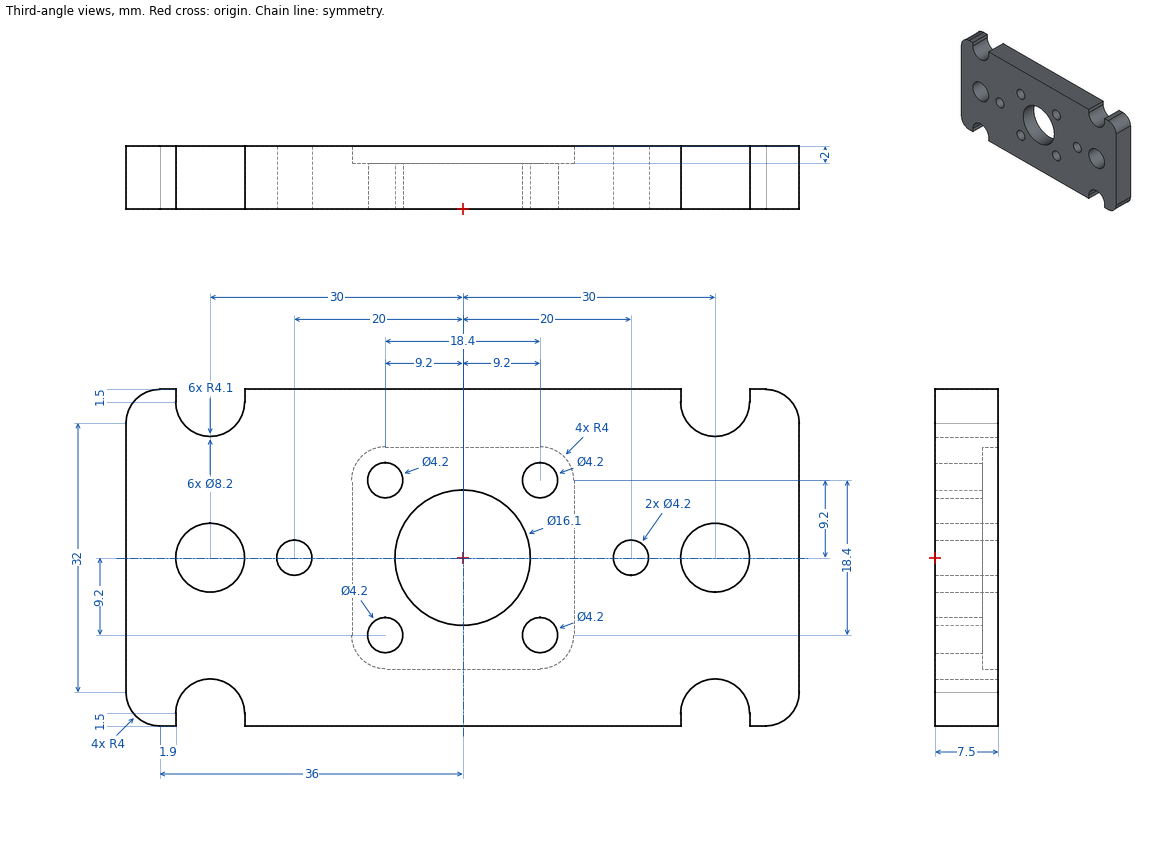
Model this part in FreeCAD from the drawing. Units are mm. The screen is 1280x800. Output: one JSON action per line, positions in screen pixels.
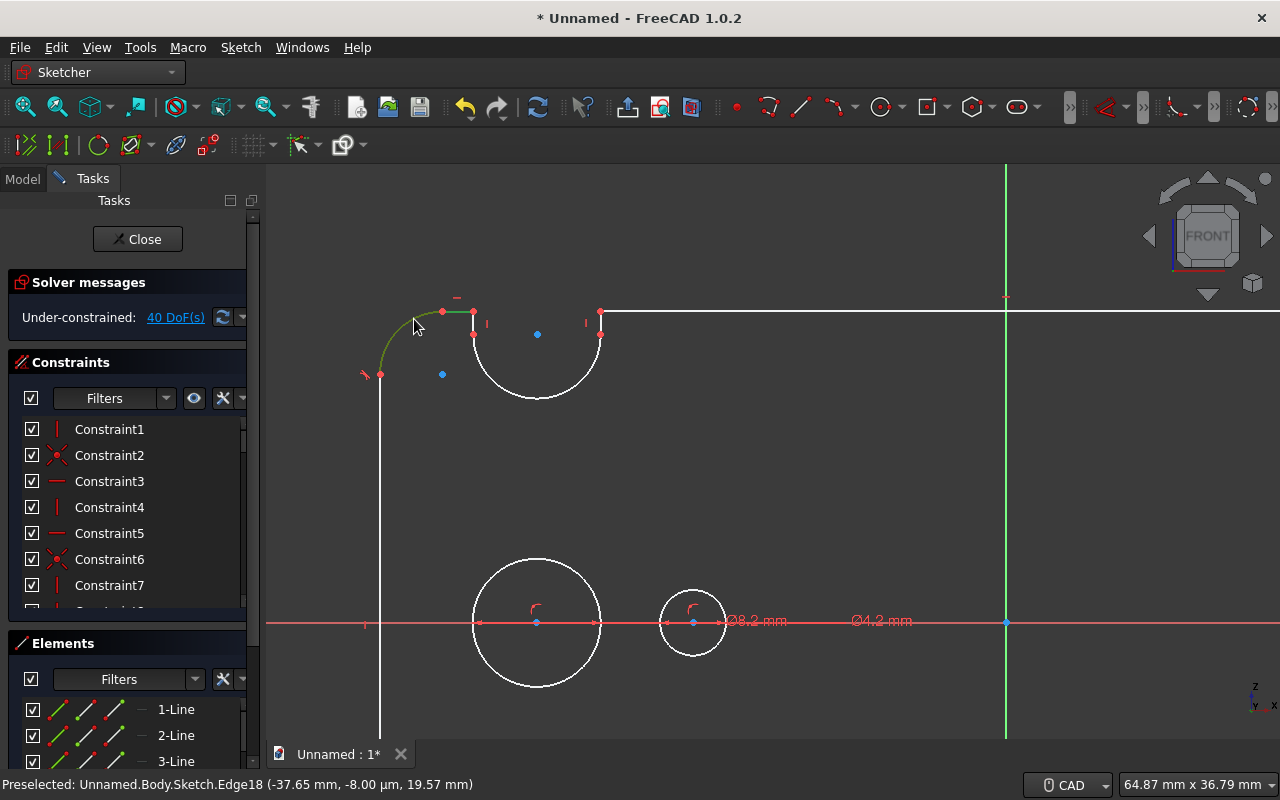
{"action": "key", "text": "t"}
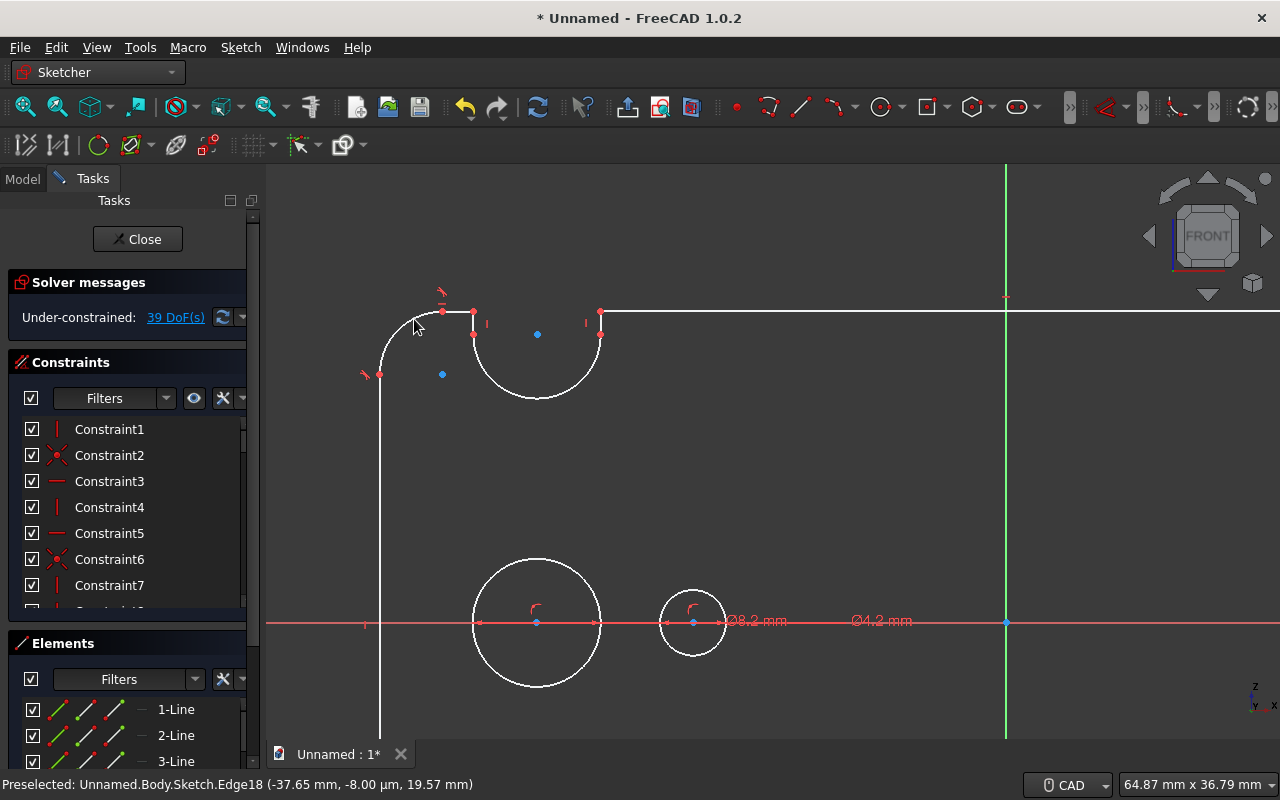
{"action": "scroll", "coordinate": [473, 321], "scroll_direction": "up", "scroll_amount": 3}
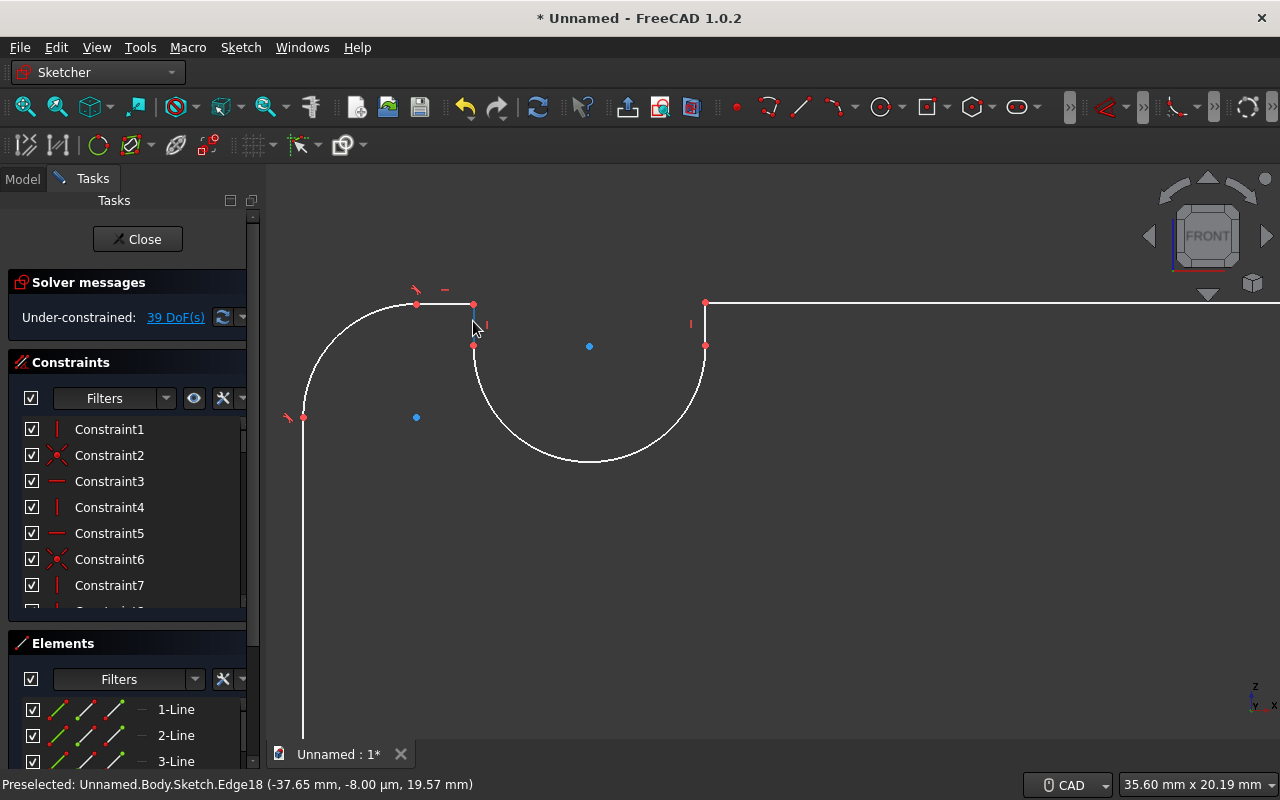
{"action": "left_click", "coordinate": [474, 320]}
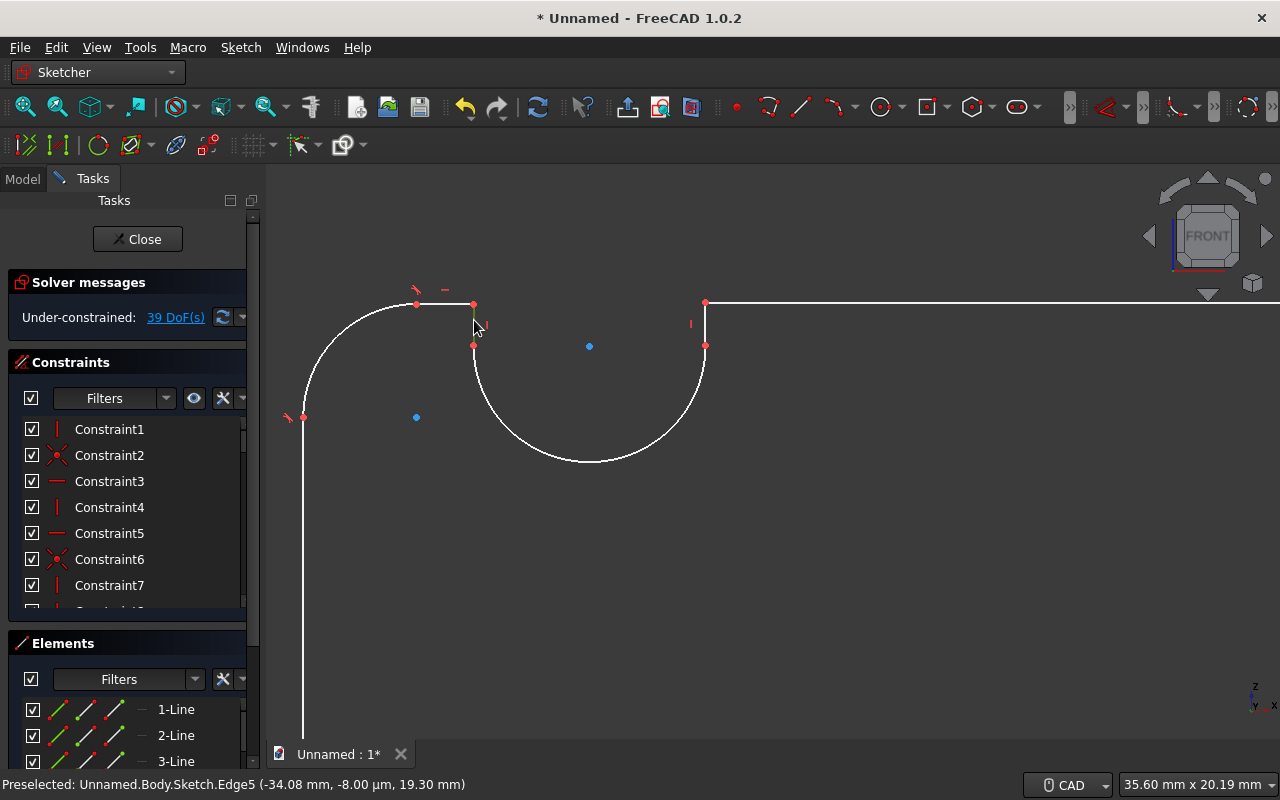
{"action": "scroll", "coordinate": [462, 314], "scroll_direction": "down", "scroll_amount": 7}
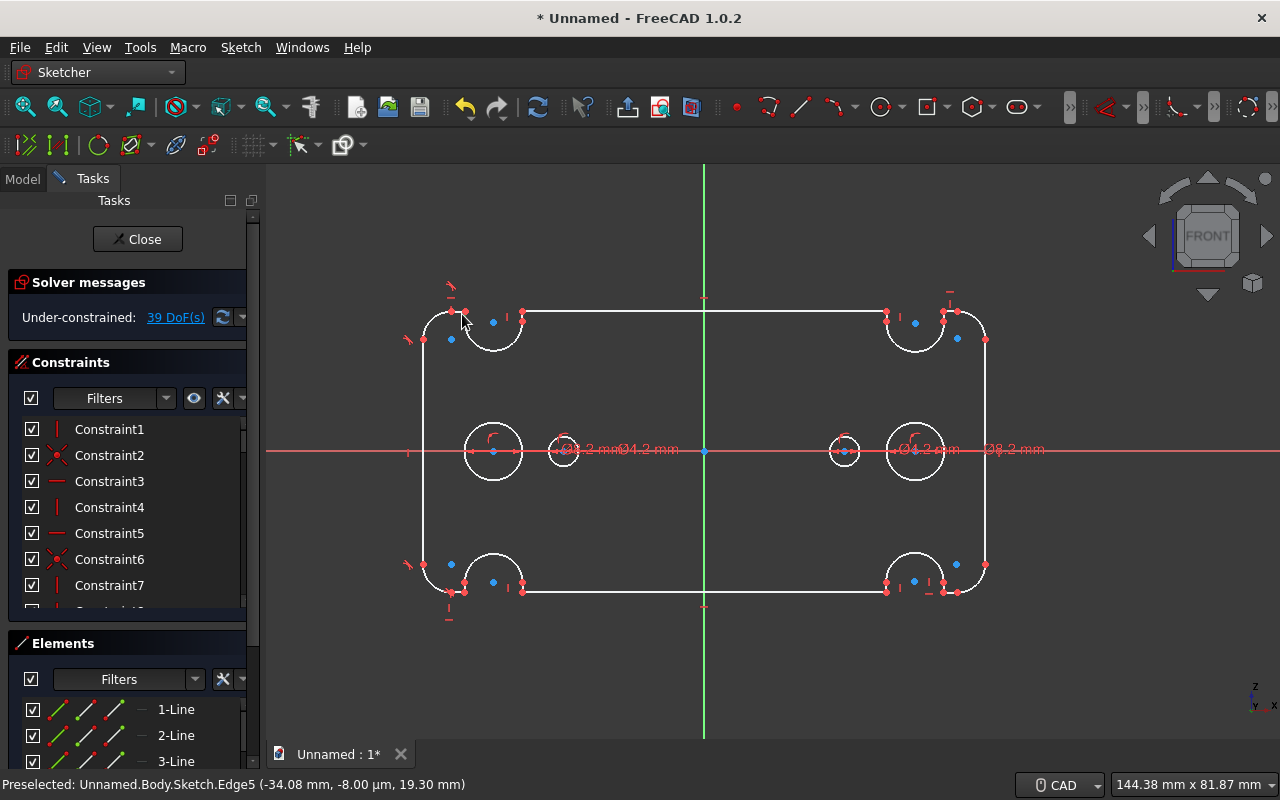
{"action": "left_click", "coordinate": [477, 345]}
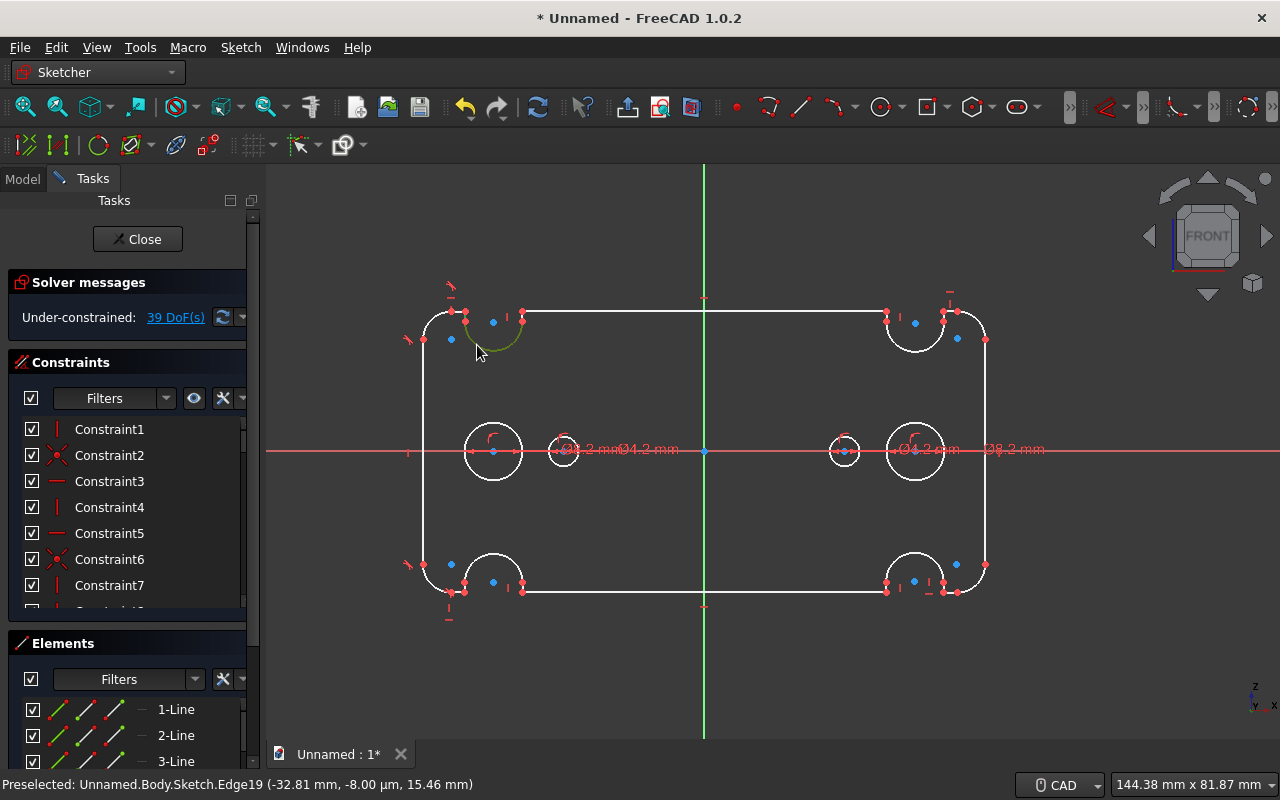
{"action": "key", "text": "t"}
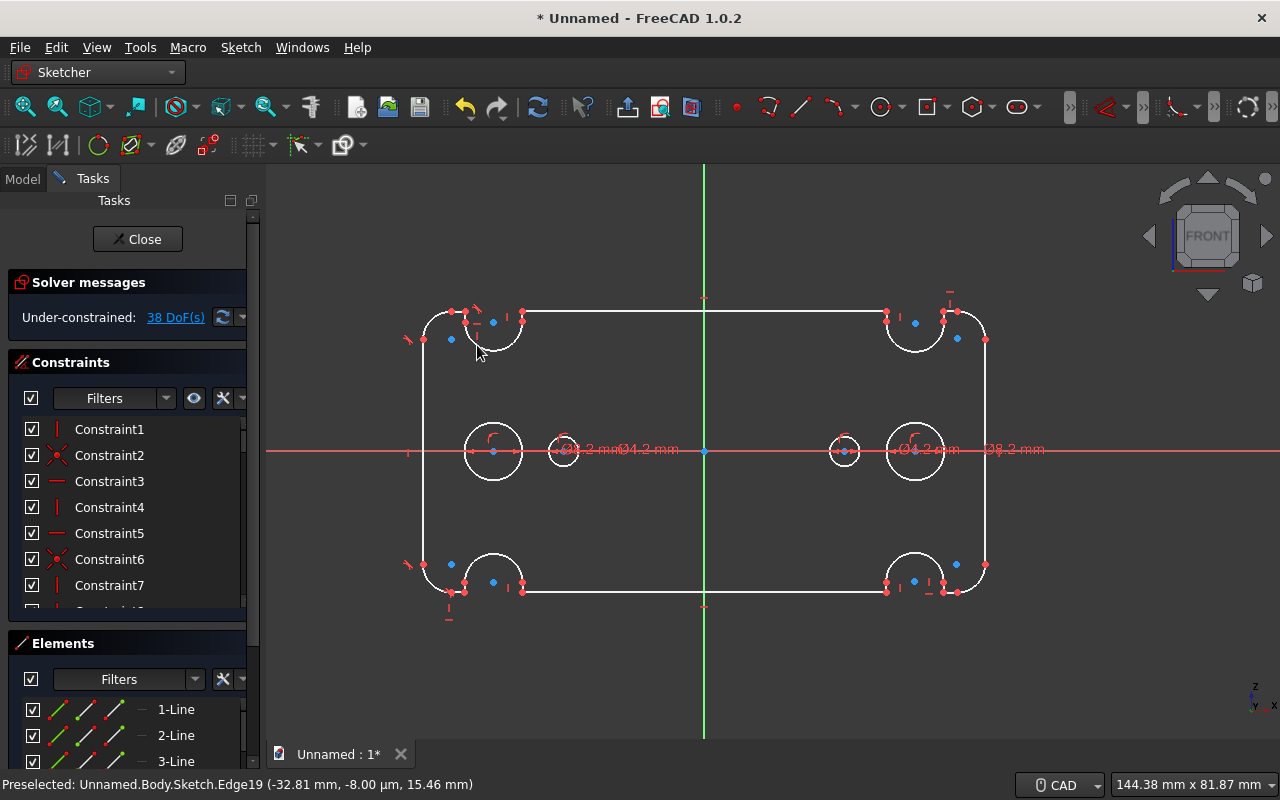
{"action": "scroll", "coordinate": [522, 317], "scroll_direction": "up", "scroll_amount": 5}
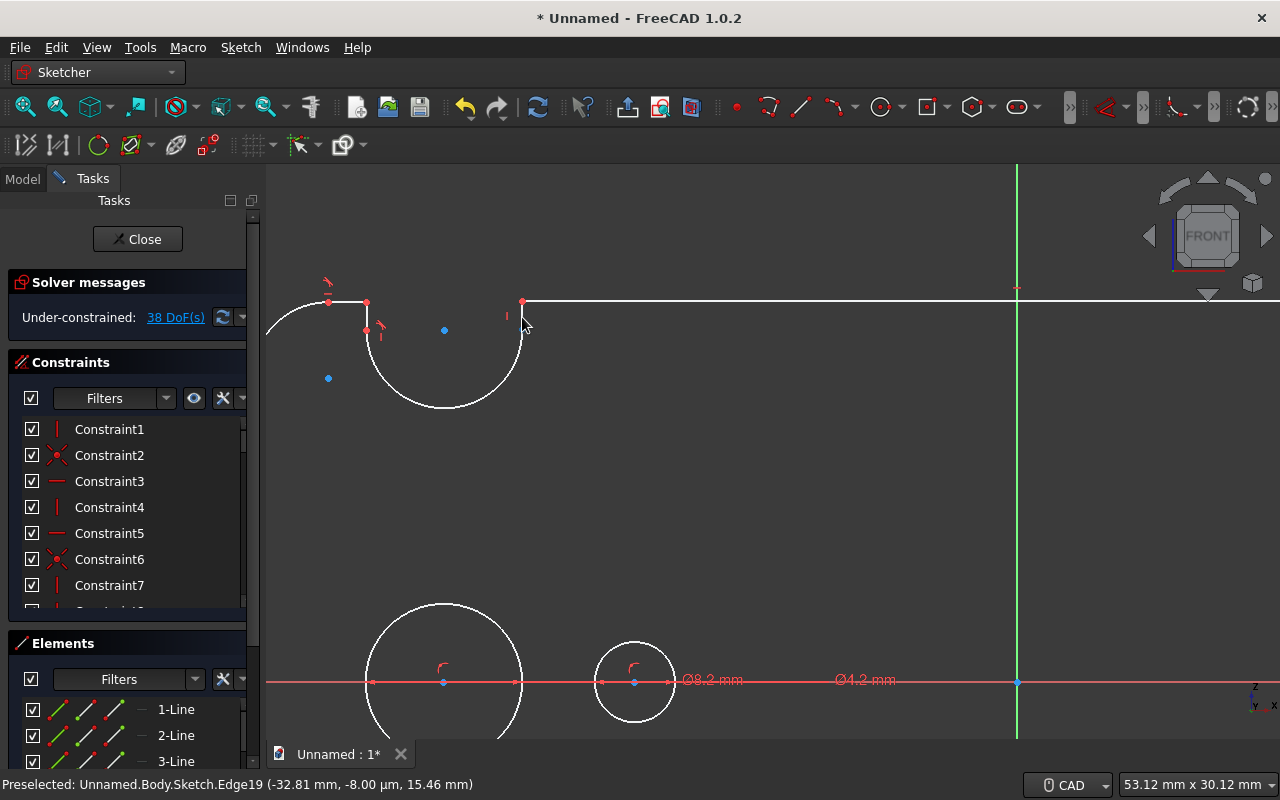
{"action": "left_click", "coordinate": [522, 316]}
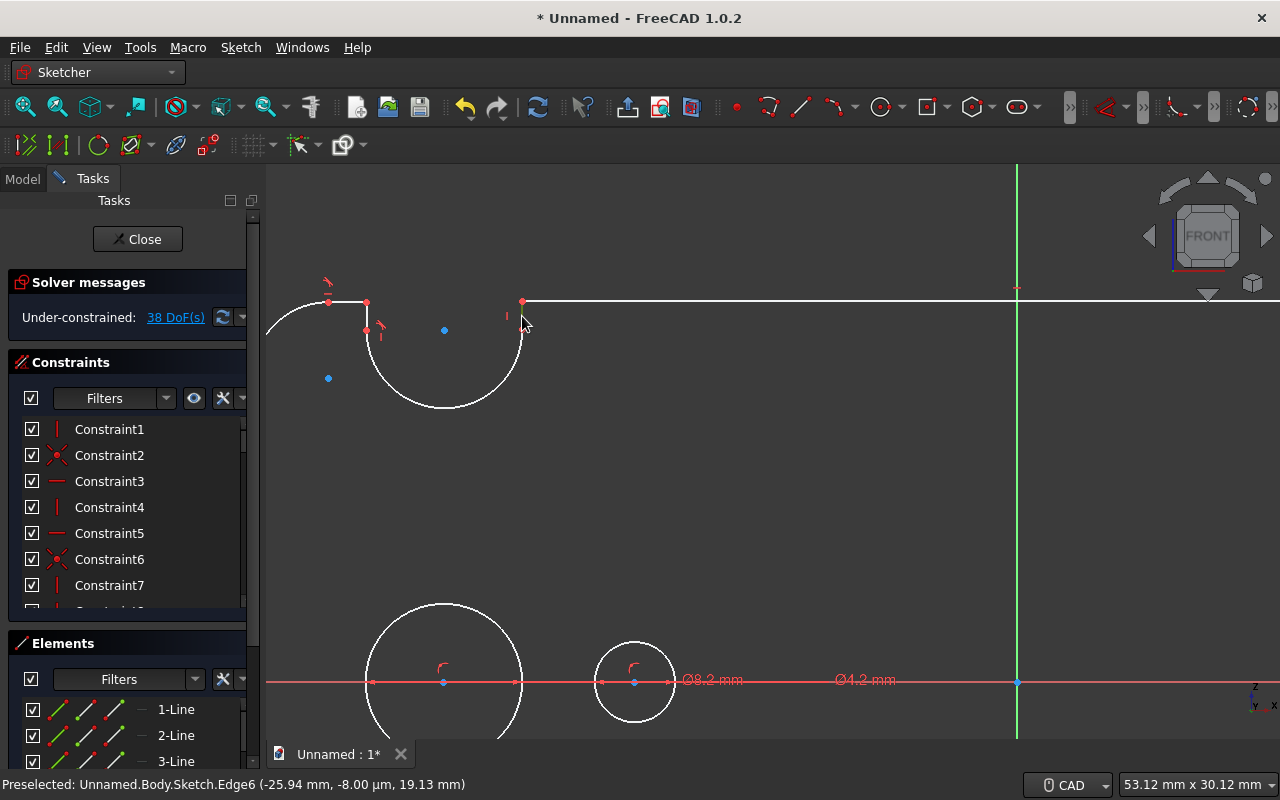
{"action": "left_click", "coordinate": [399, 394]}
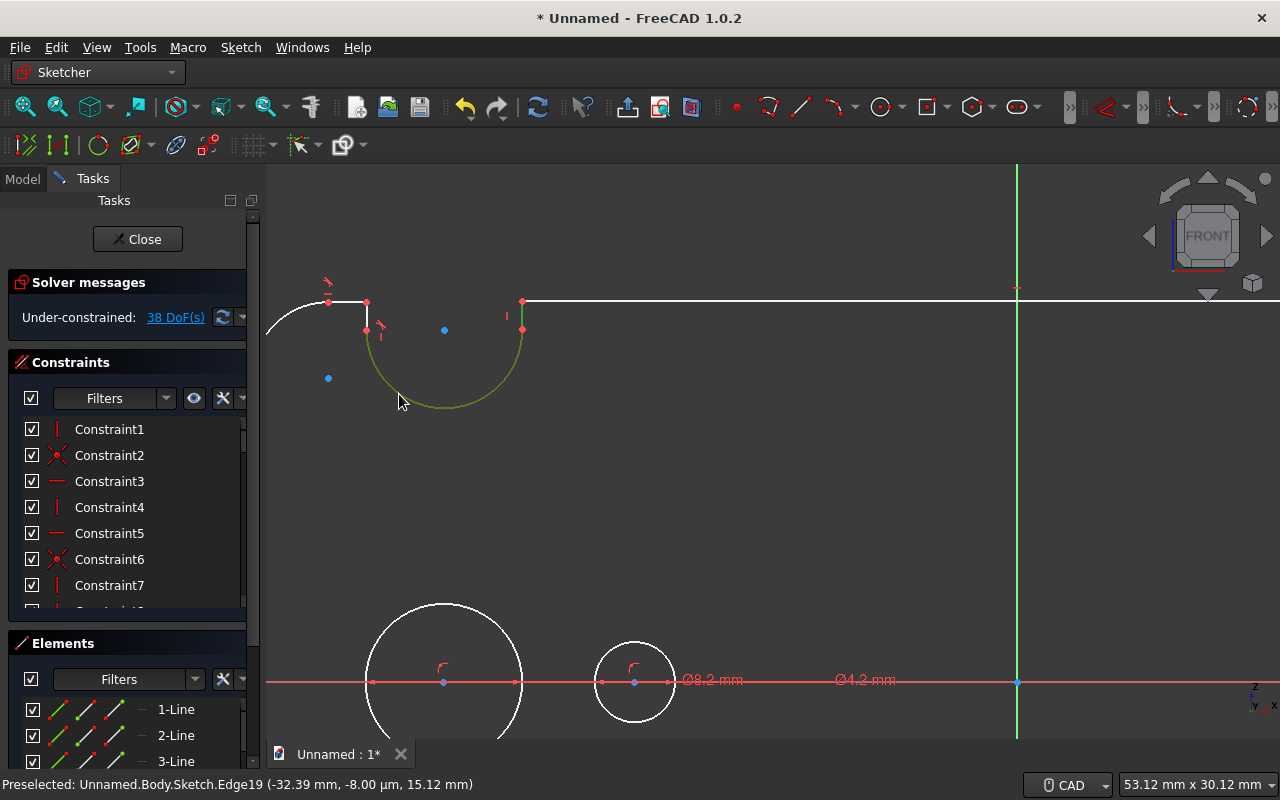
{"action": "key", "text": "t"}